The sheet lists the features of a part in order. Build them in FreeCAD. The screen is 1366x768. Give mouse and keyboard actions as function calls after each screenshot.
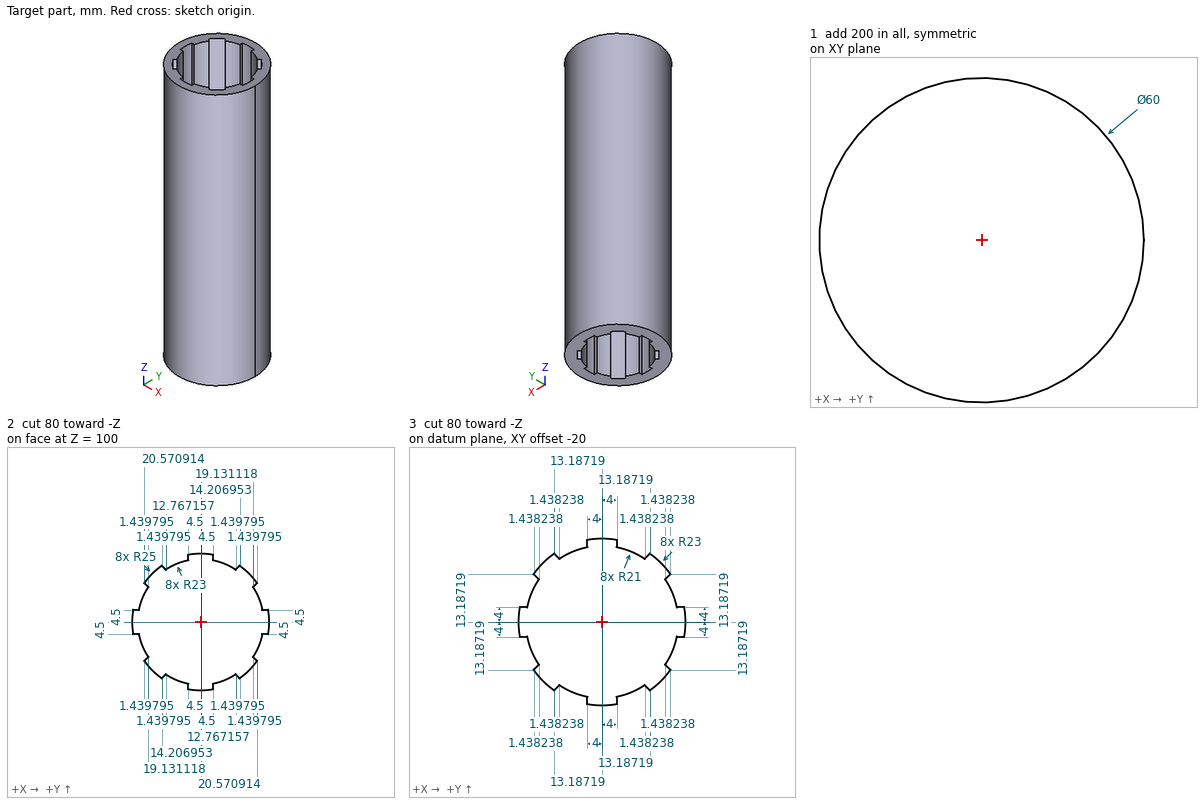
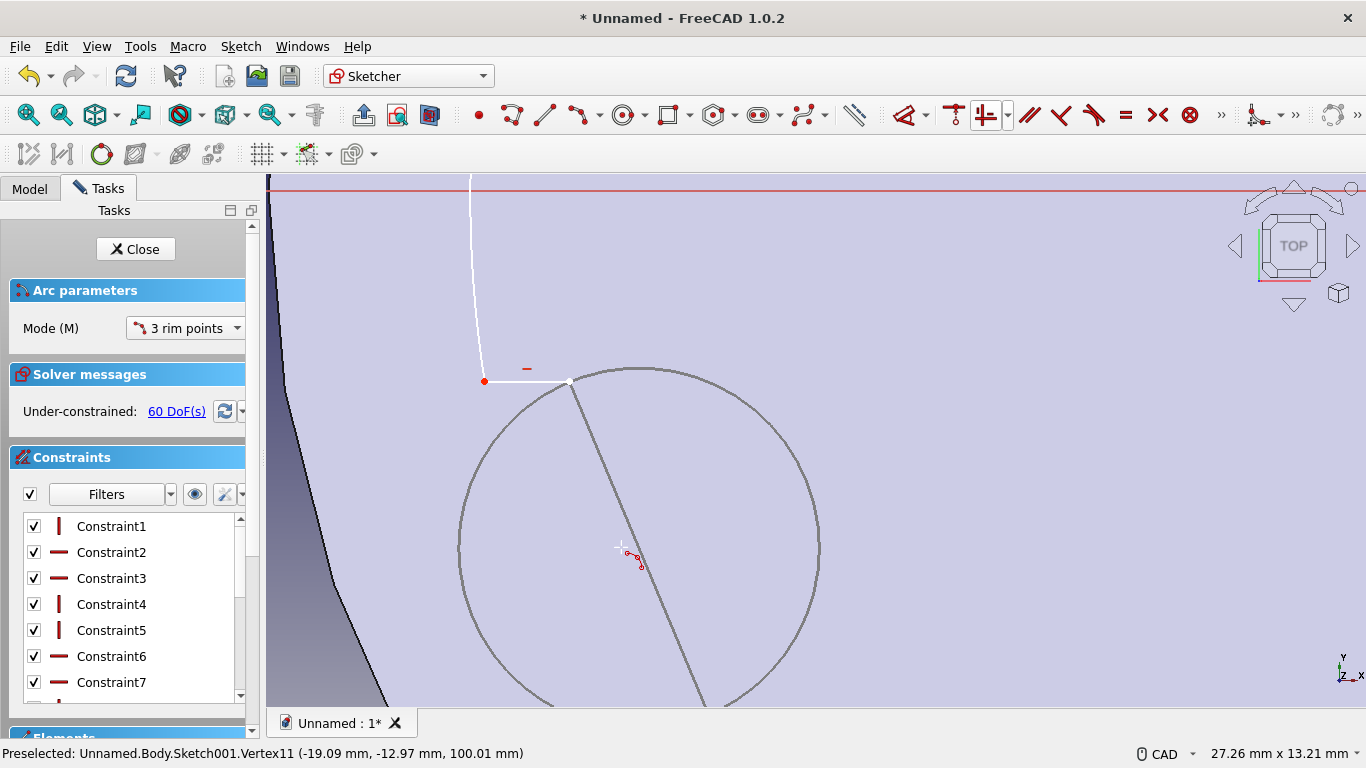
click(622, 547)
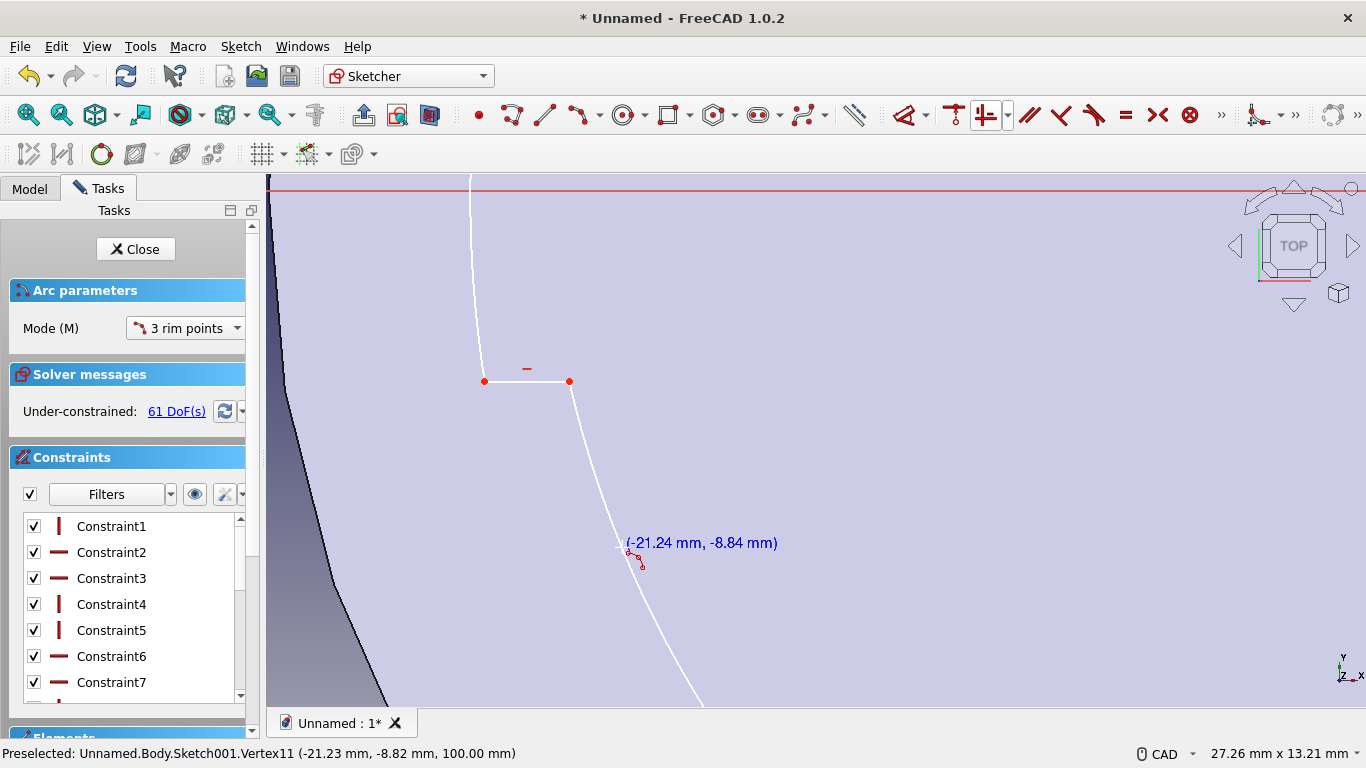
scroll(603, 490, down, 9)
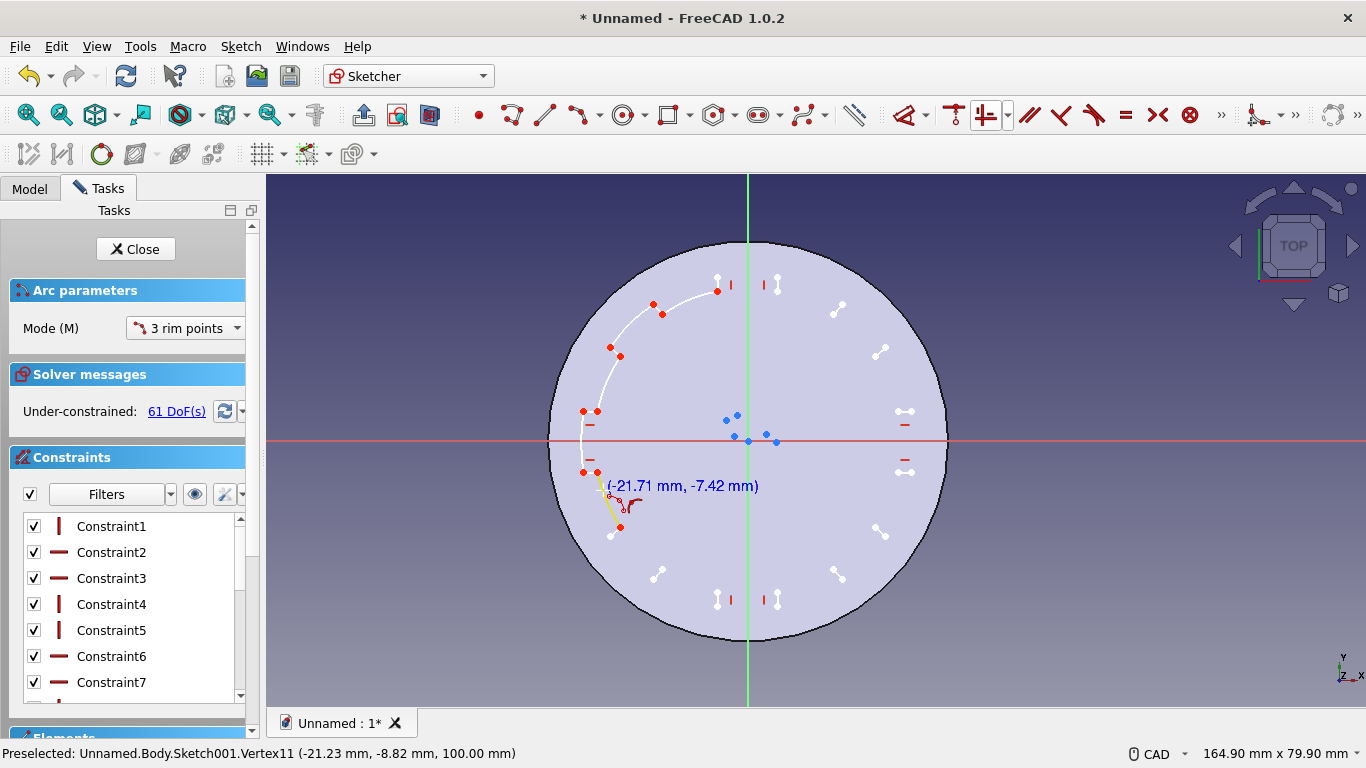
scroll(611, 536, up, 5)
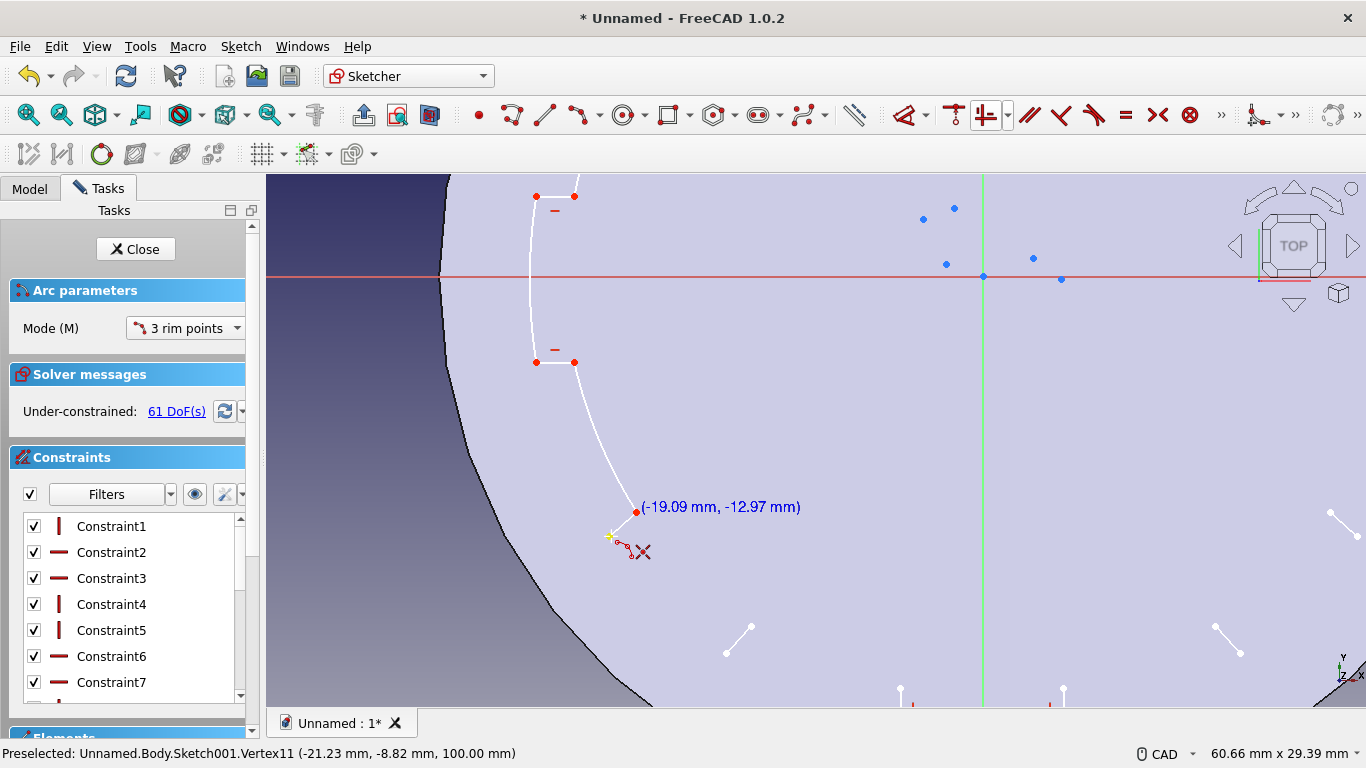
click(610, 537)
click(727, 653)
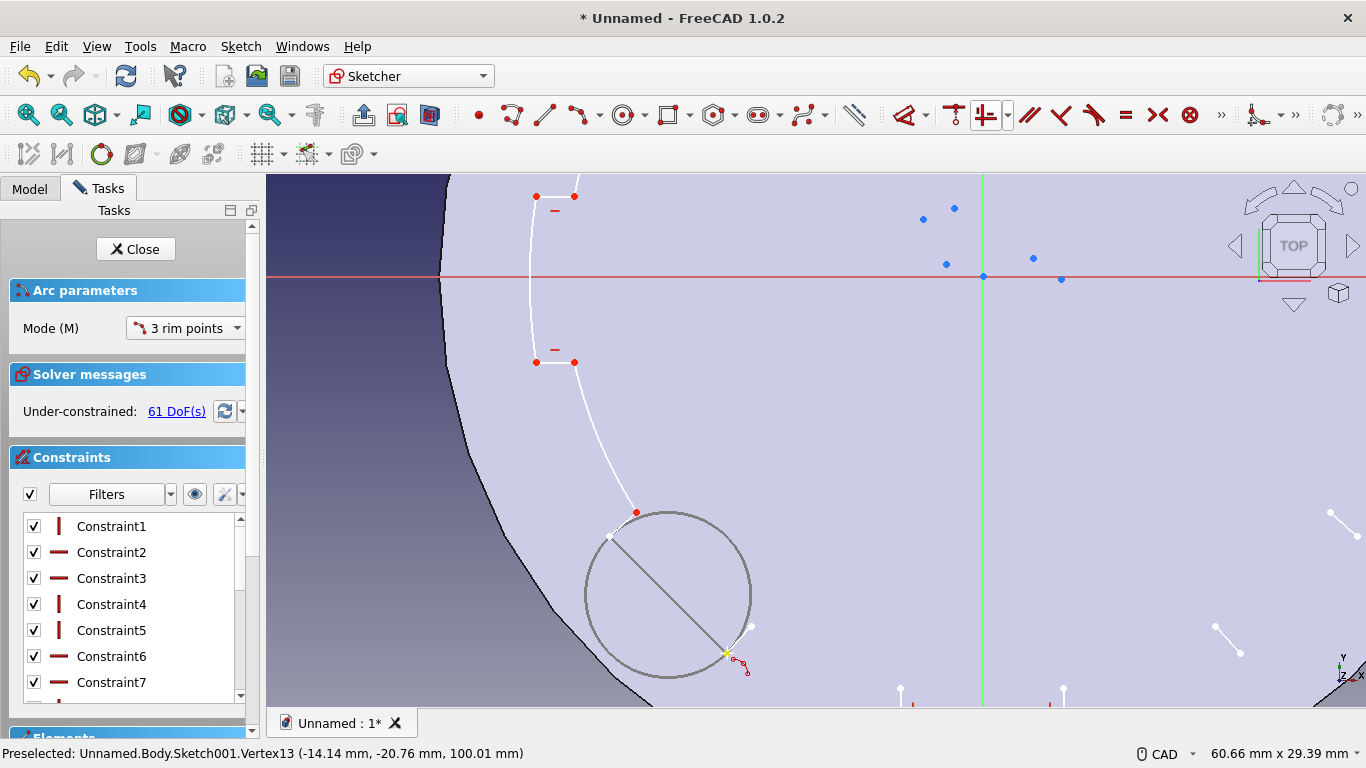
scroll(663, 598, up, 4)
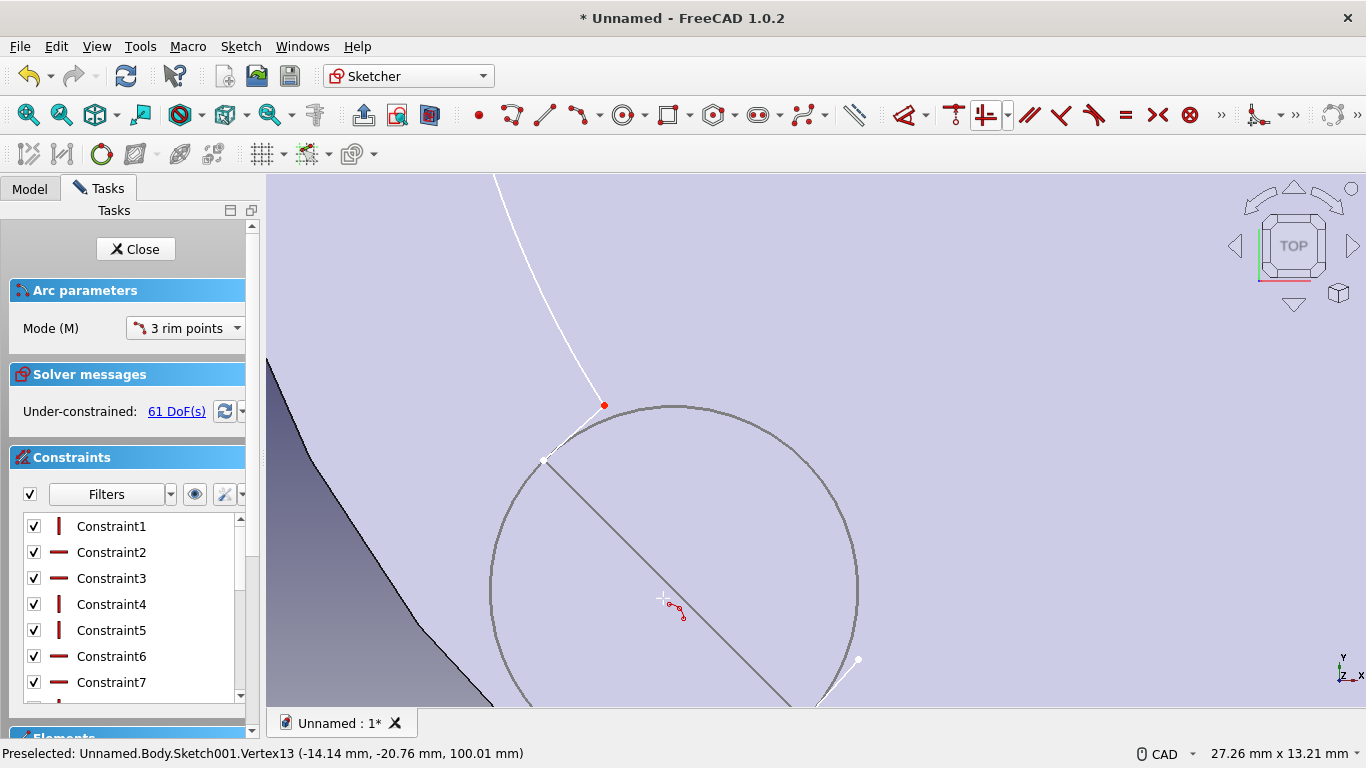
click(661, 596)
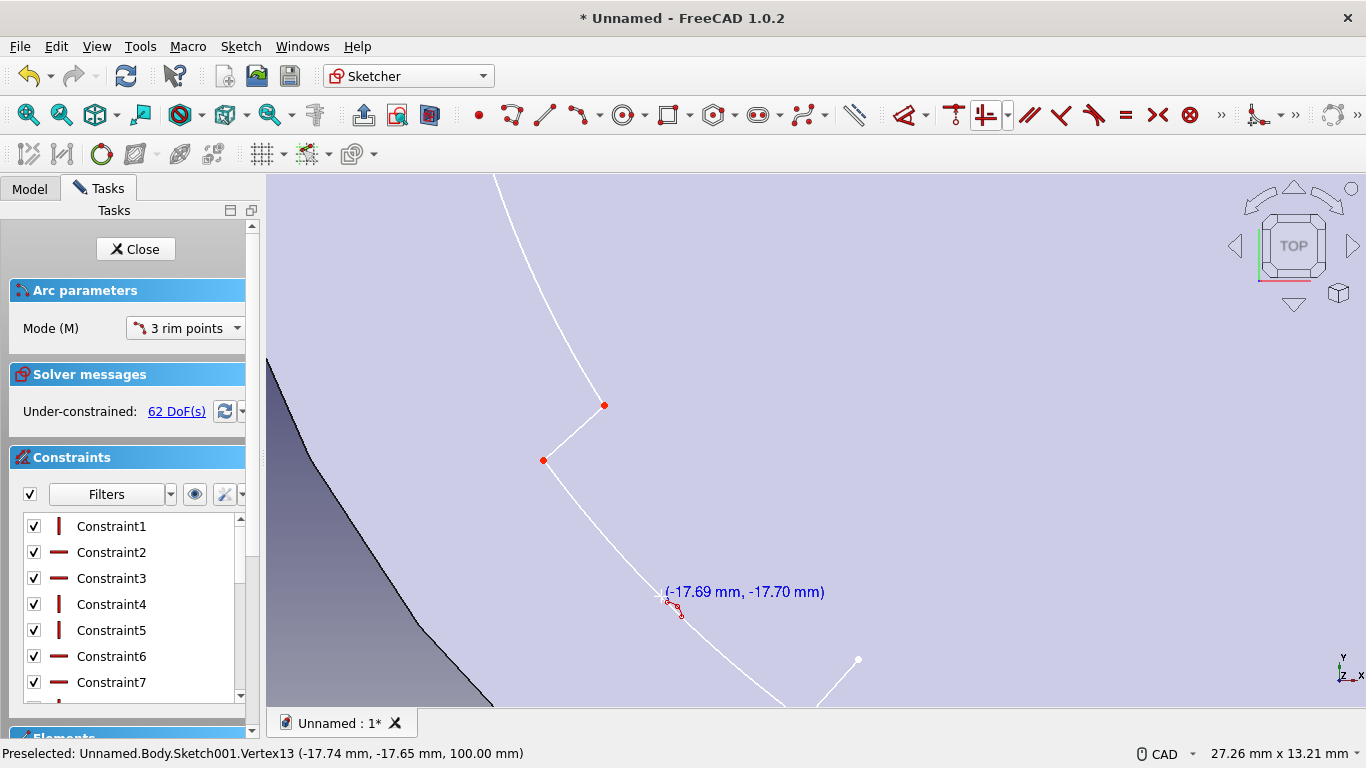
click(859, 660)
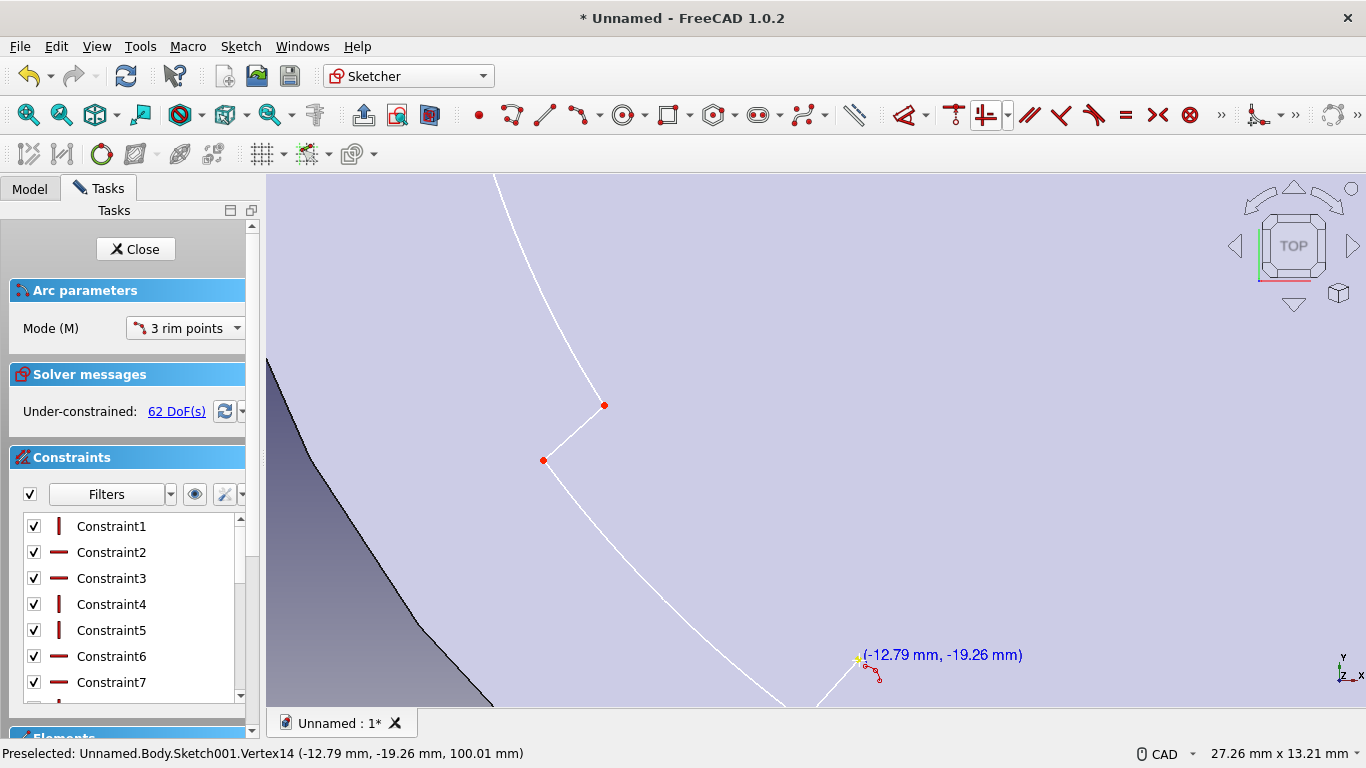
scroll(623, 551, down, 9)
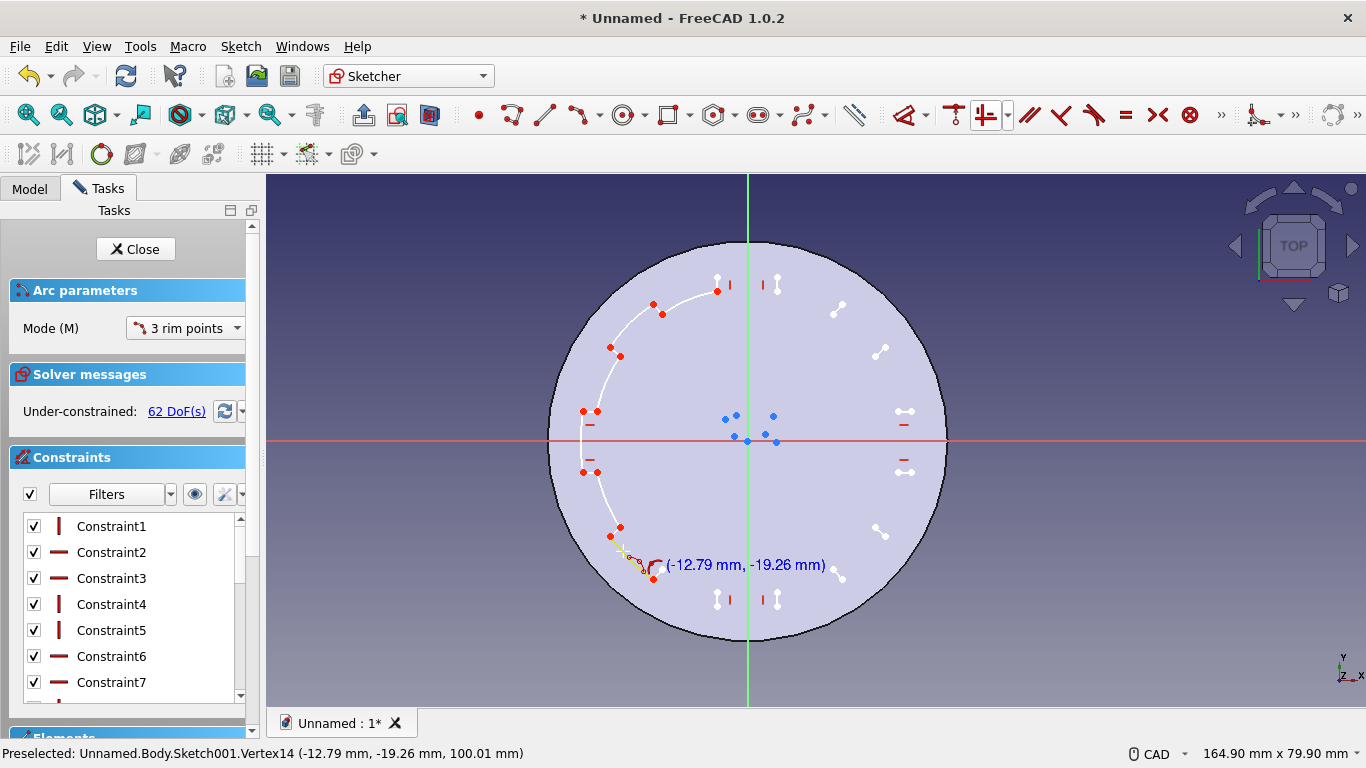
scroll(718, 592, up, 5)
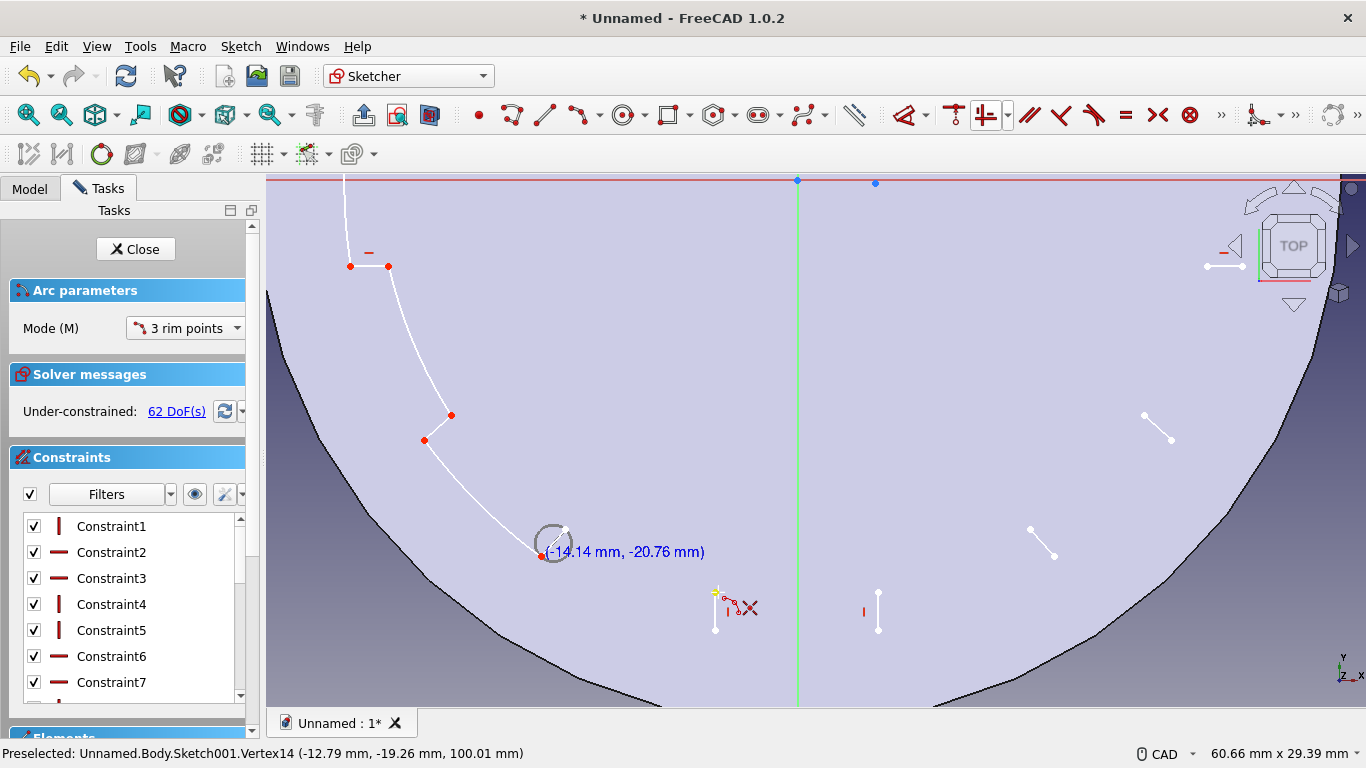
click(715, 592)